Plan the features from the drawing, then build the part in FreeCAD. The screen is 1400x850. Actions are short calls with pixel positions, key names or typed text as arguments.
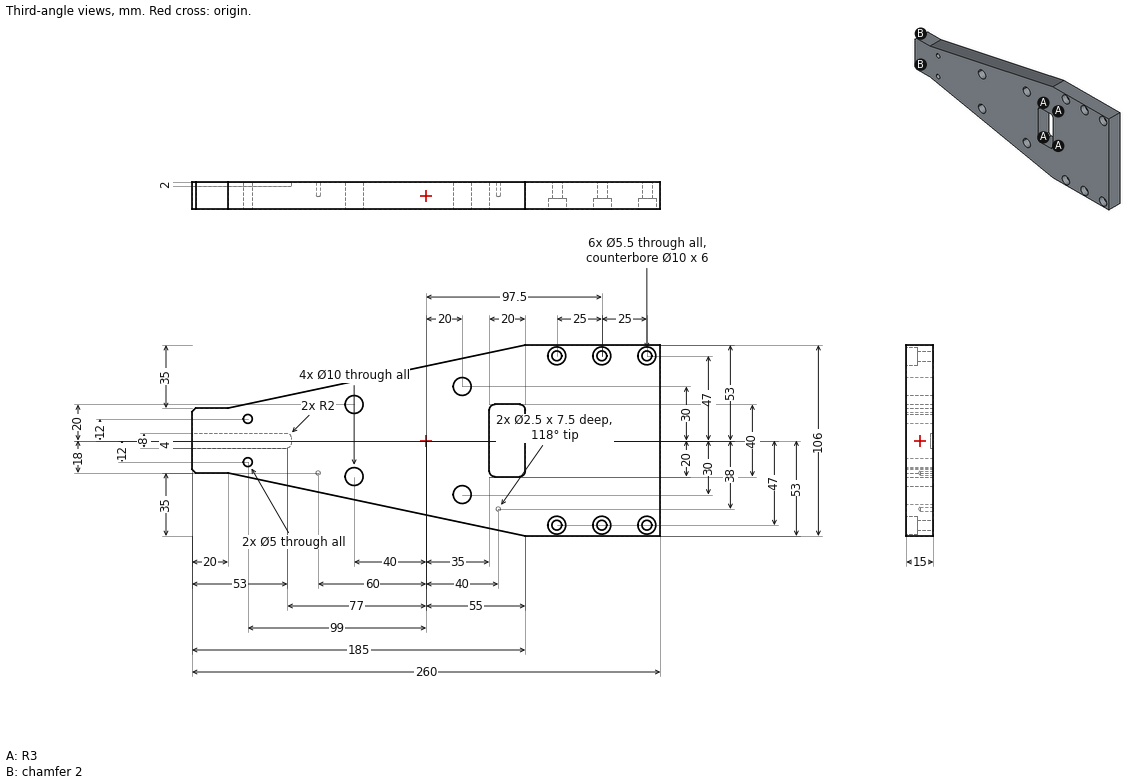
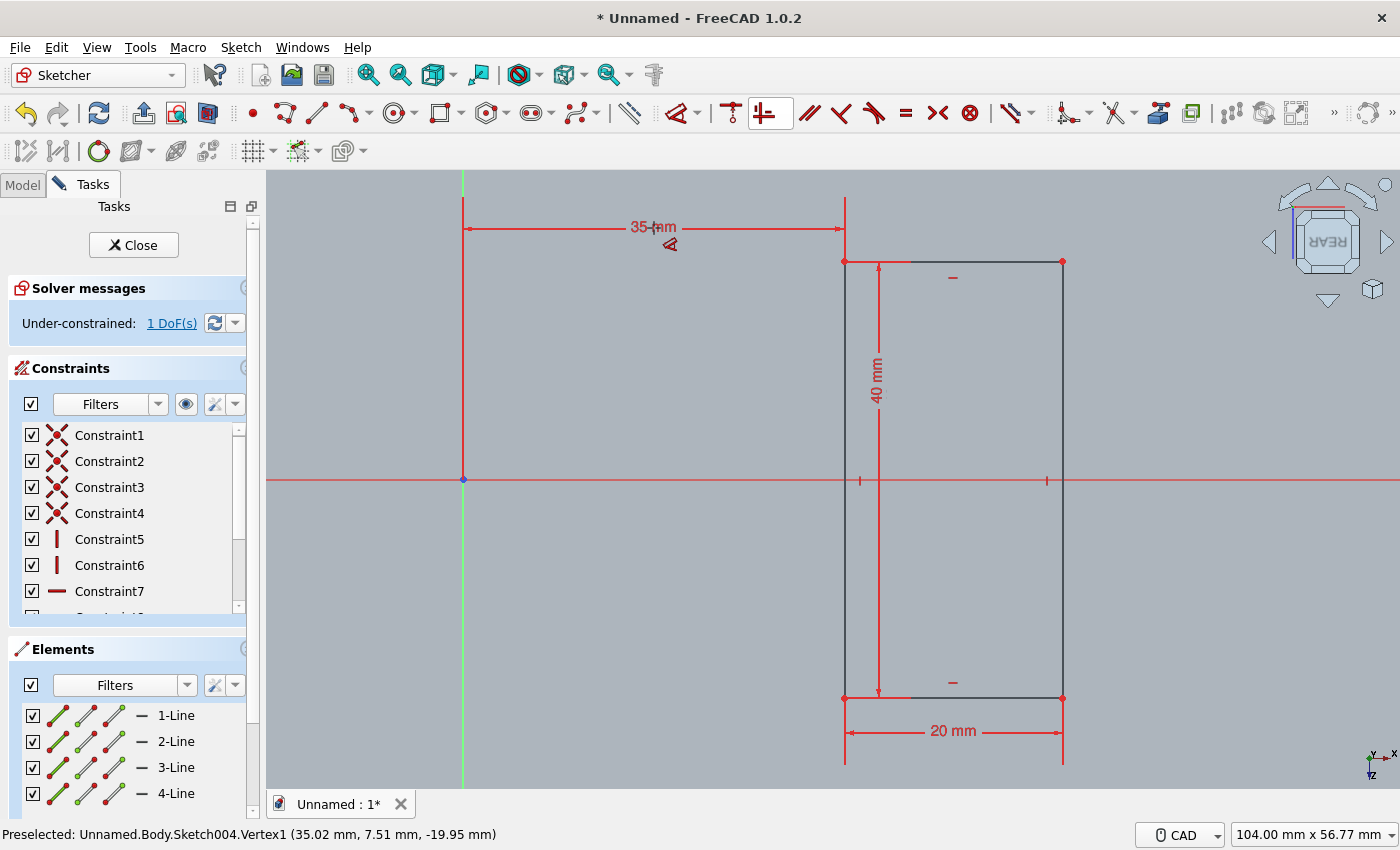
click(845, 262)
click(429, 371)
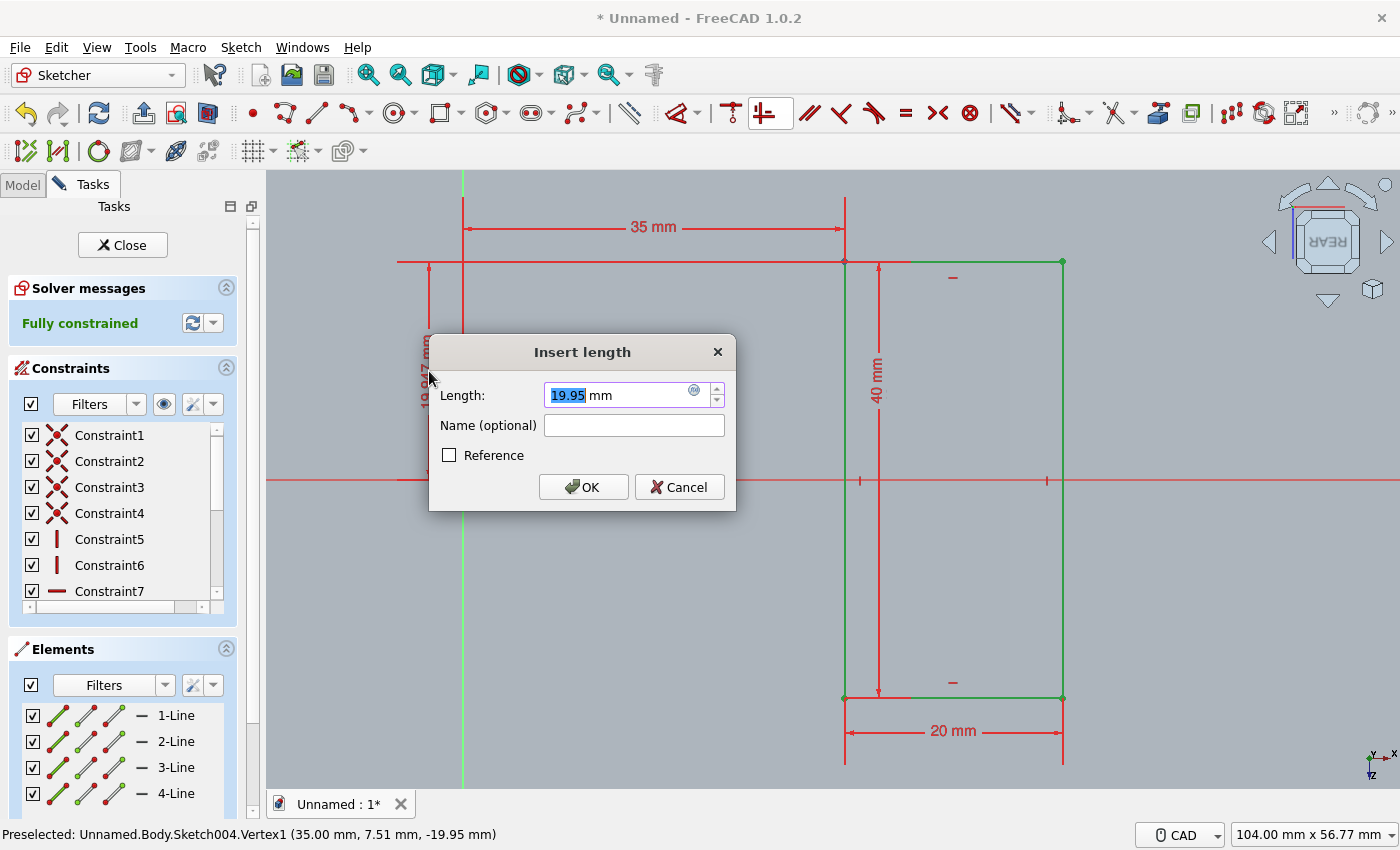
text(20)
key(Return)
key(Escape)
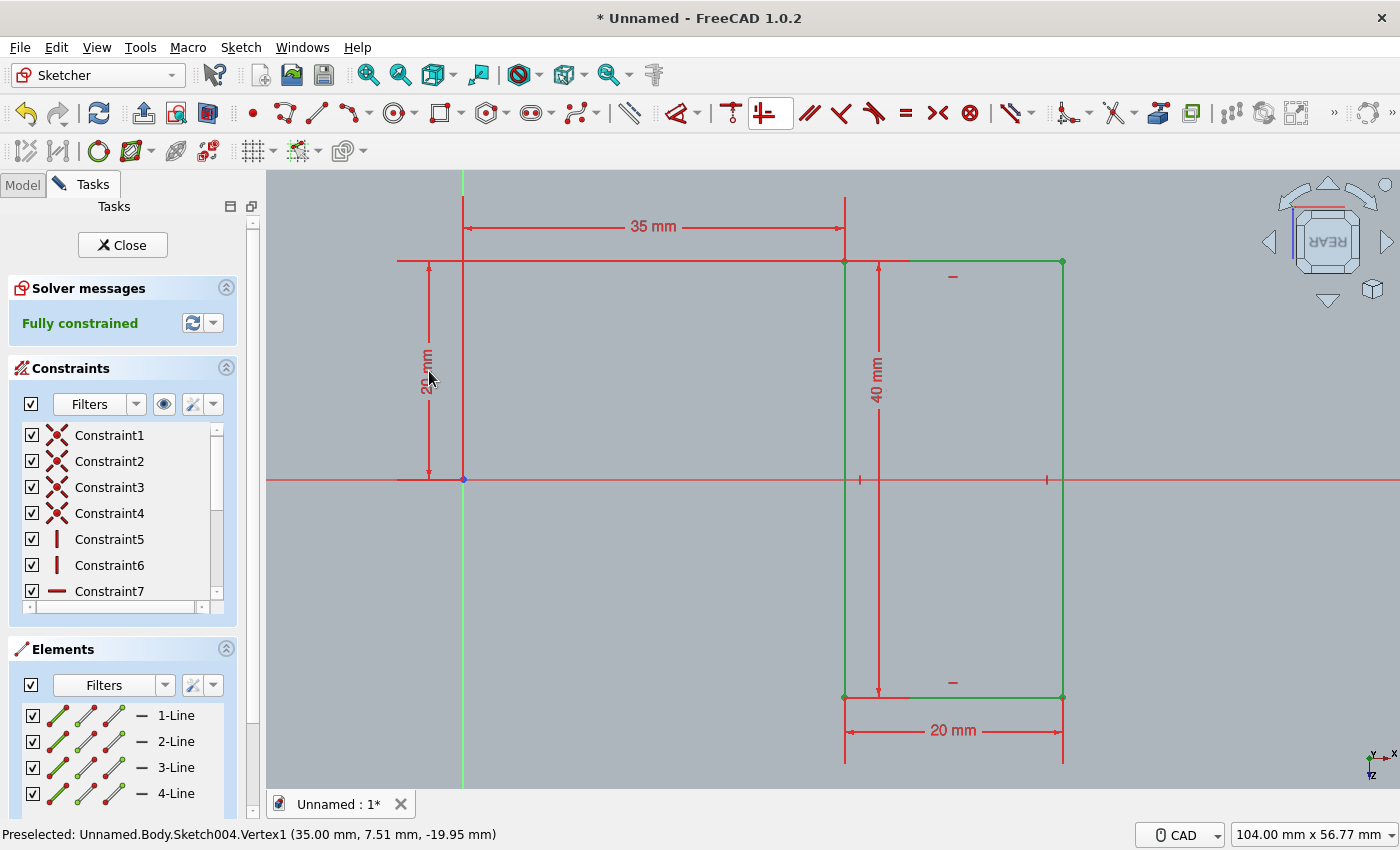
click(123, 245)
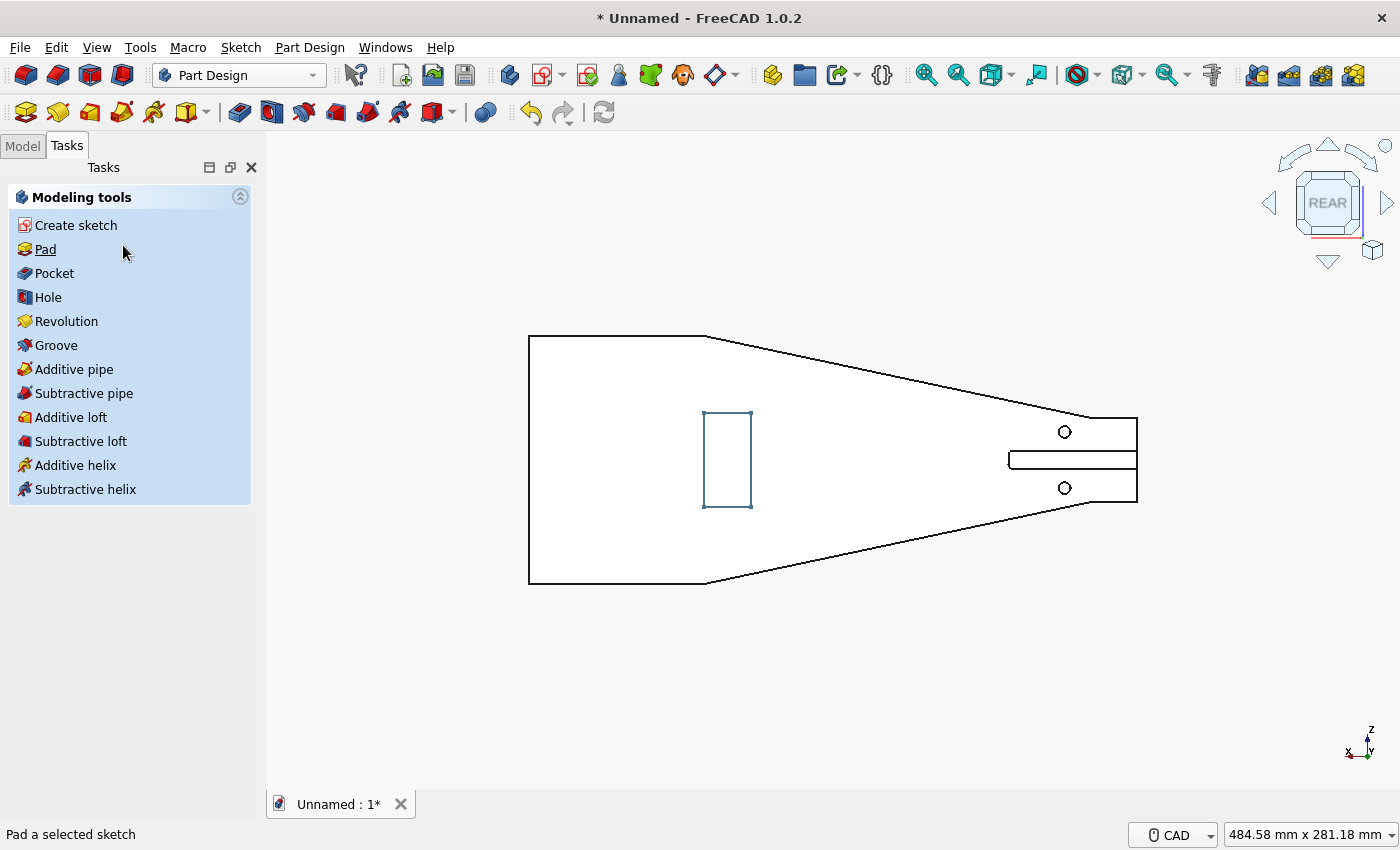
click(240, 112)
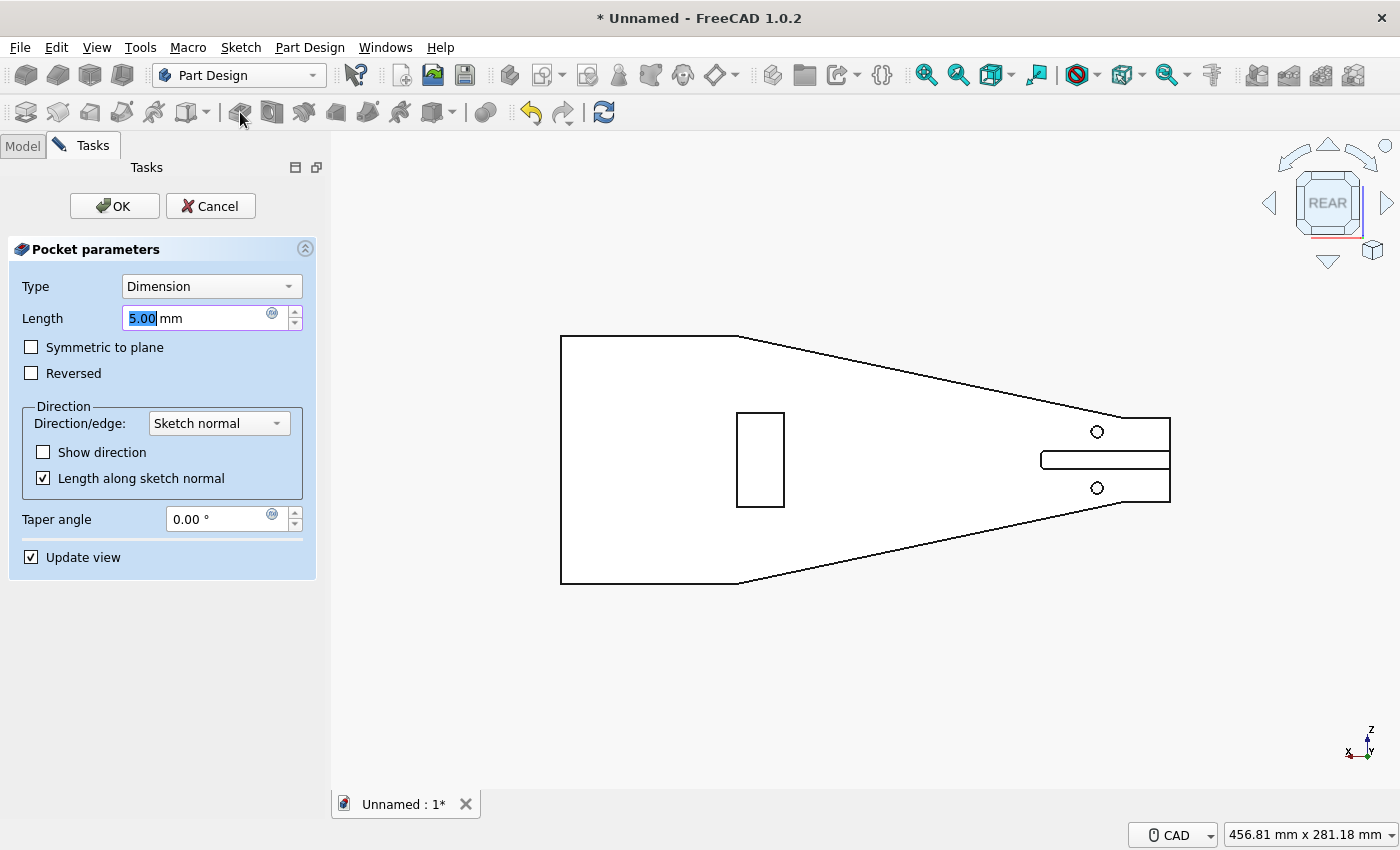
click(212, 286)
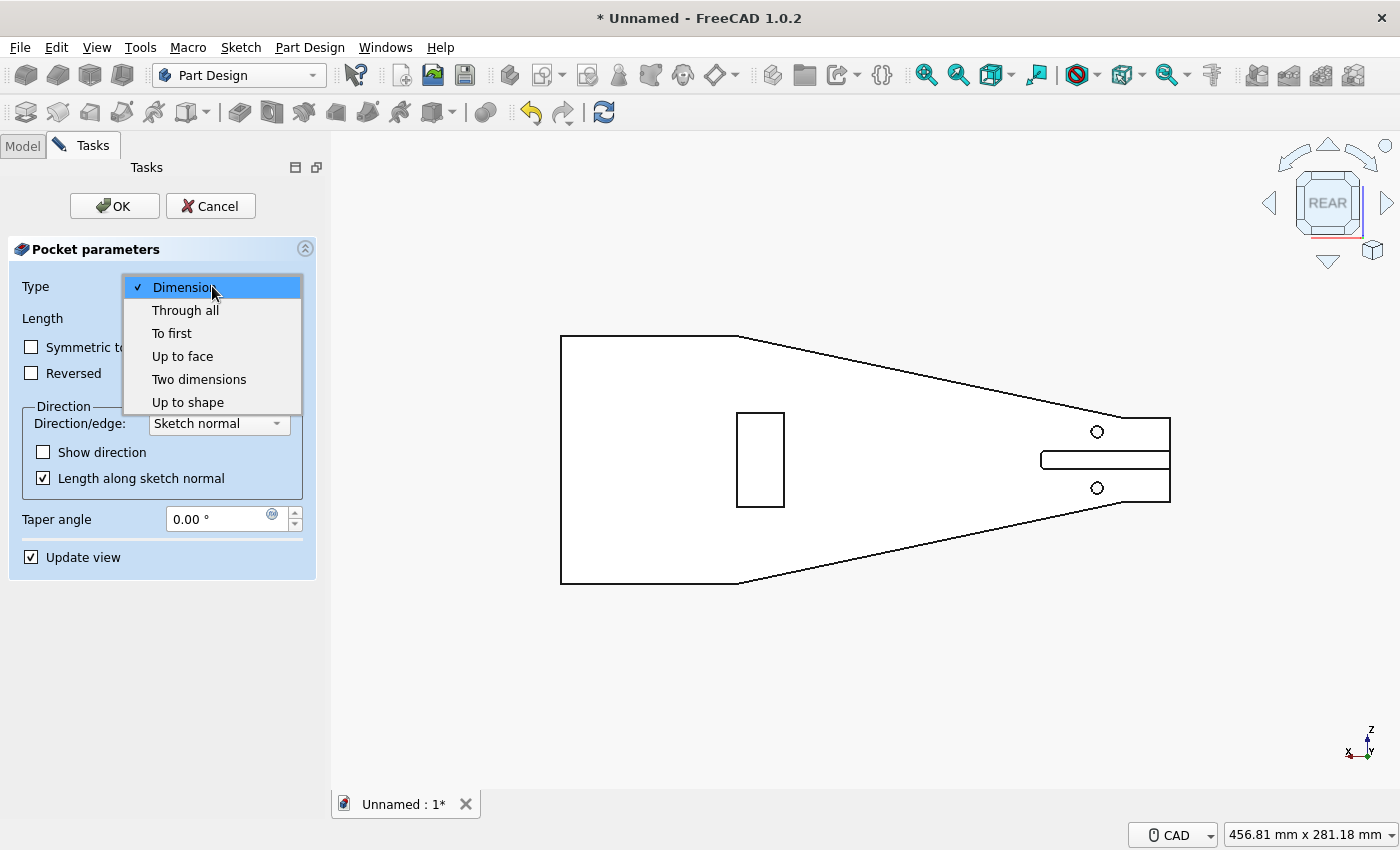
click(212, 310)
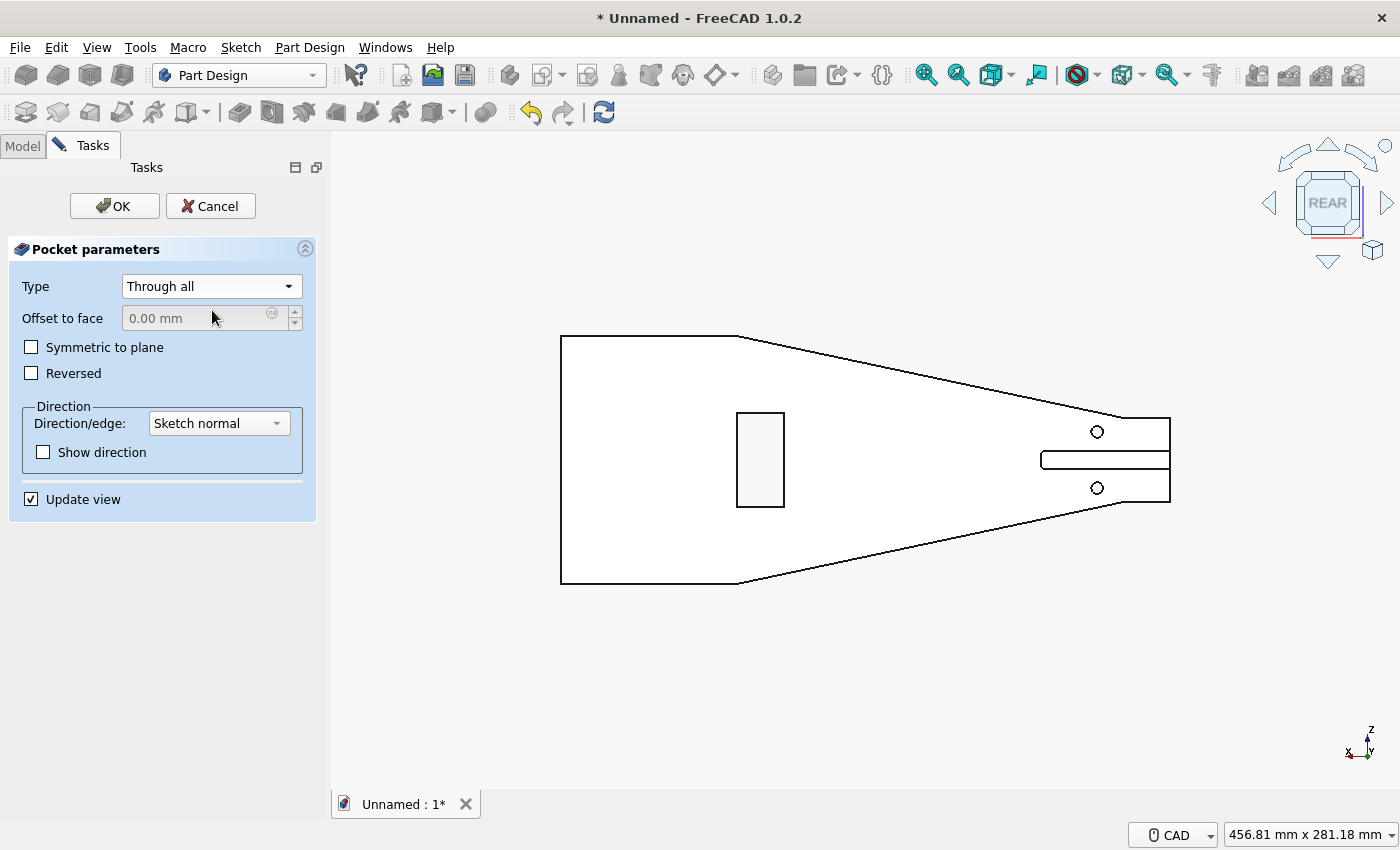
click(115, 206)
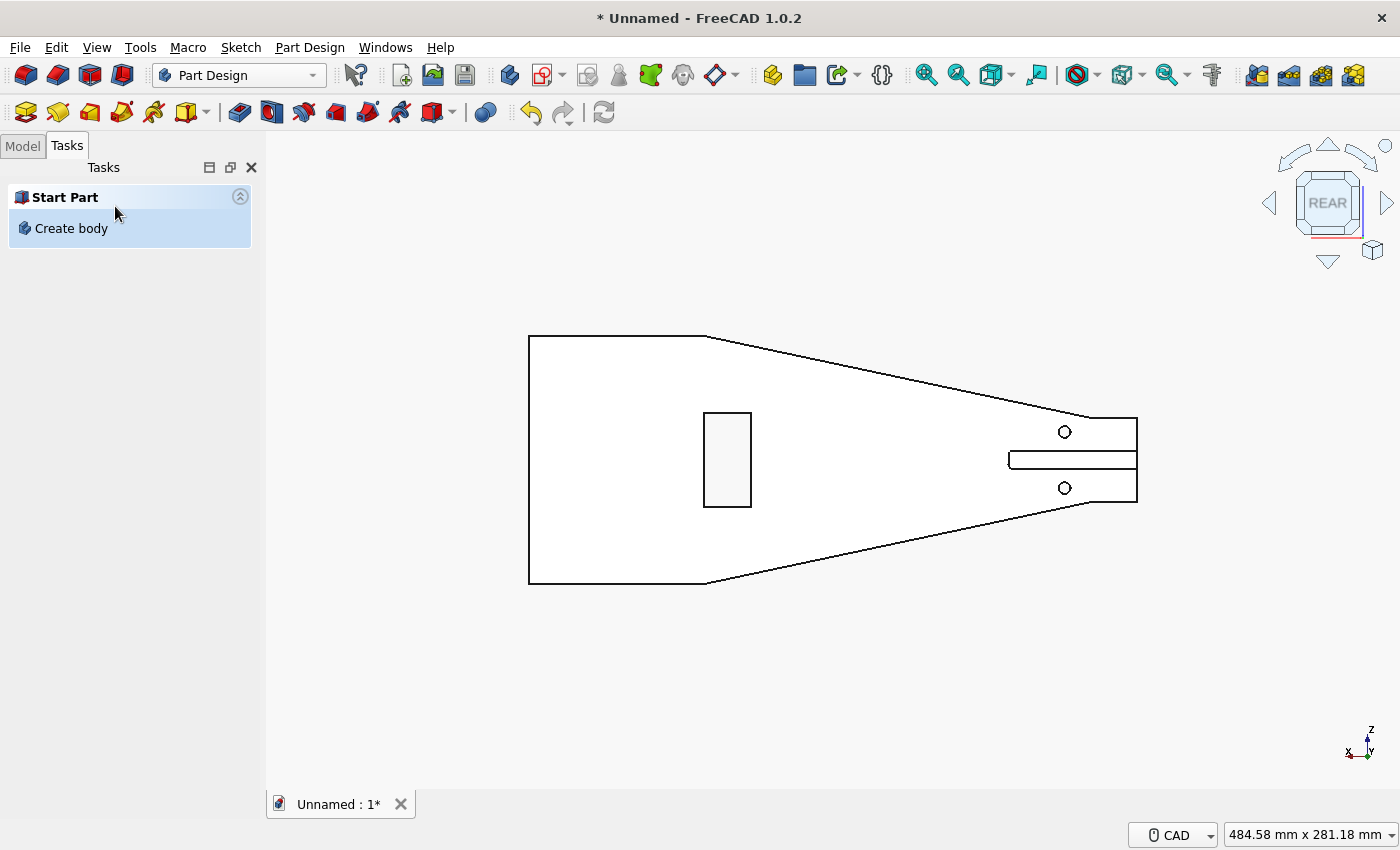
key(0)